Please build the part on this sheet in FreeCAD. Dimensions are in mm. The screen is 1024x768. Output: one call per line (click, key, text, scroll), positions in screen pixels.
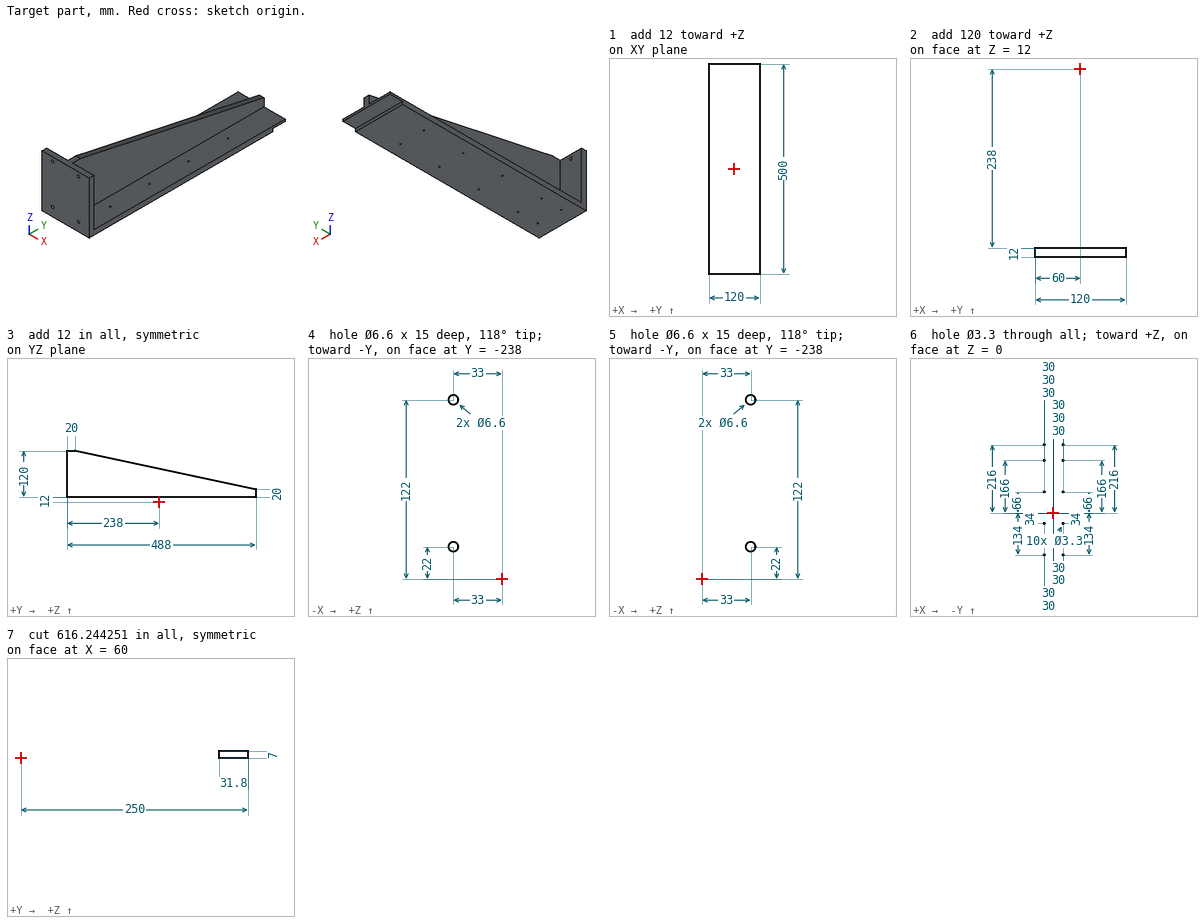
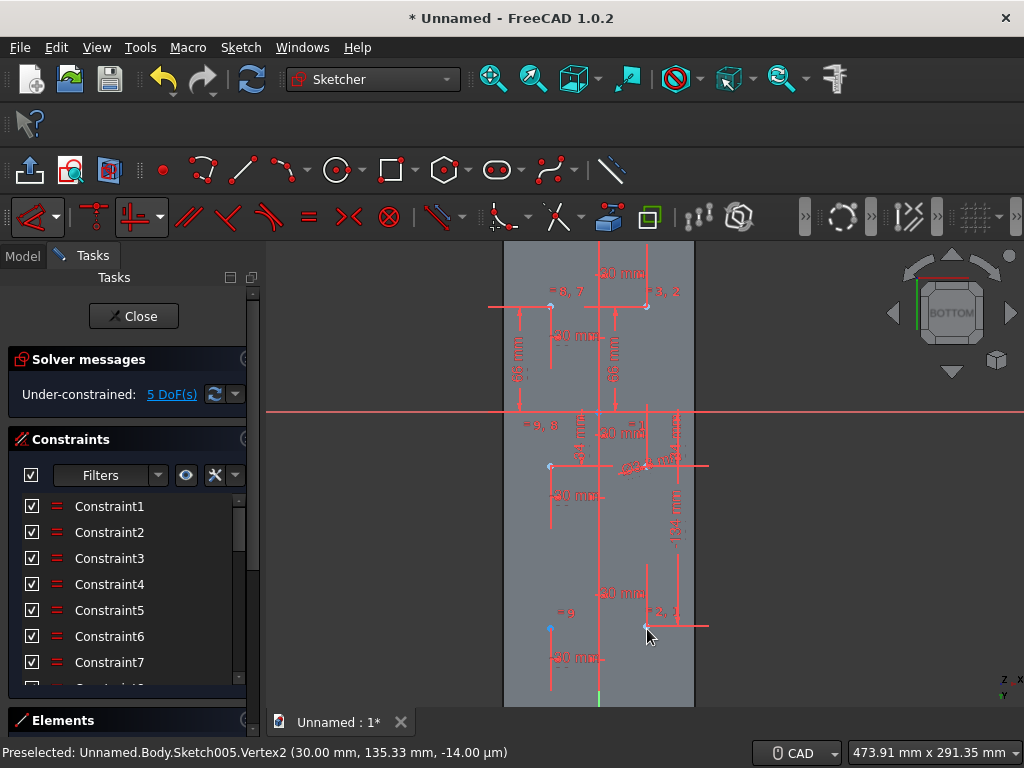
scroll(550, 629, down, 3)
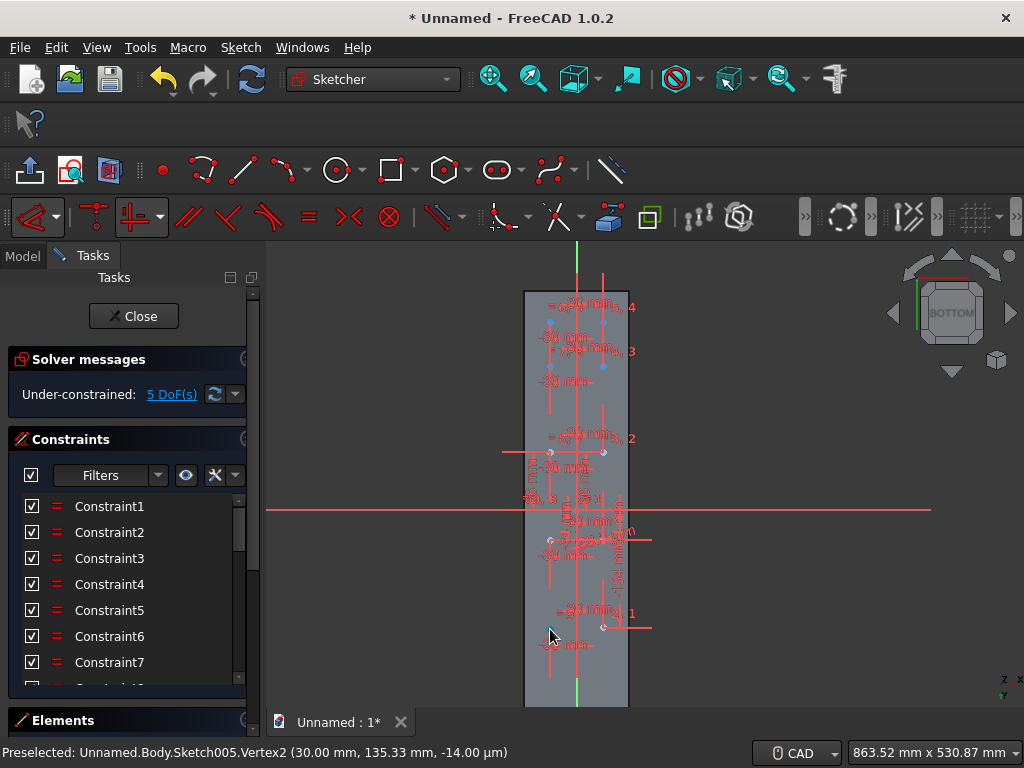
click(603, 366)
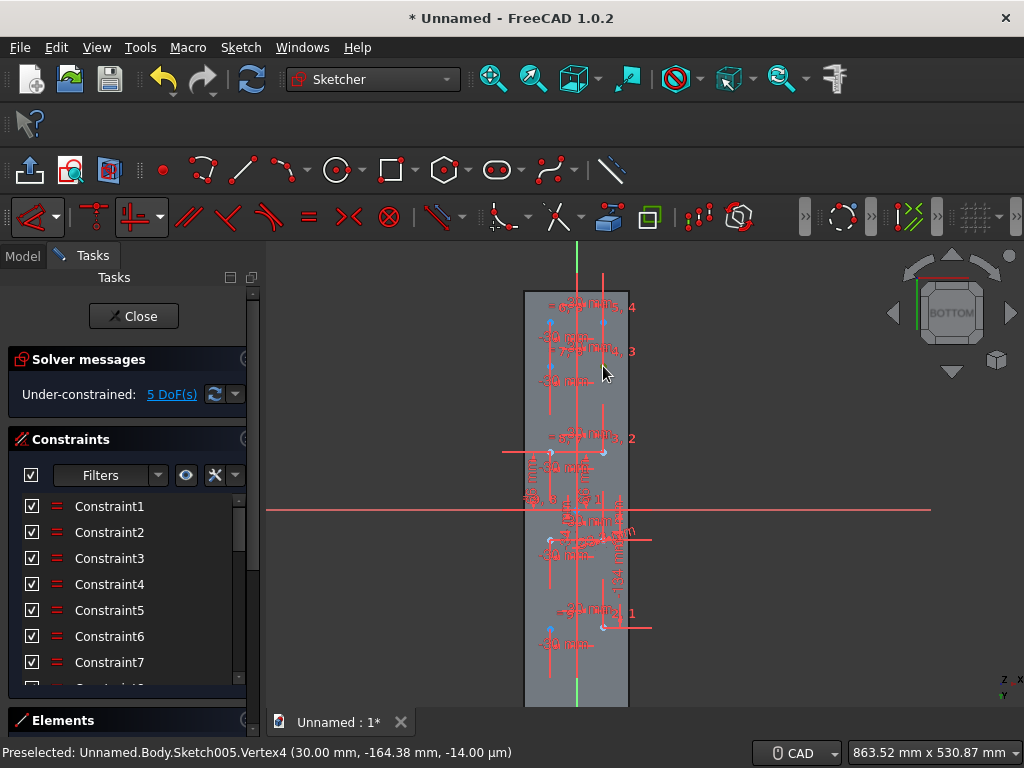
click(58, 218)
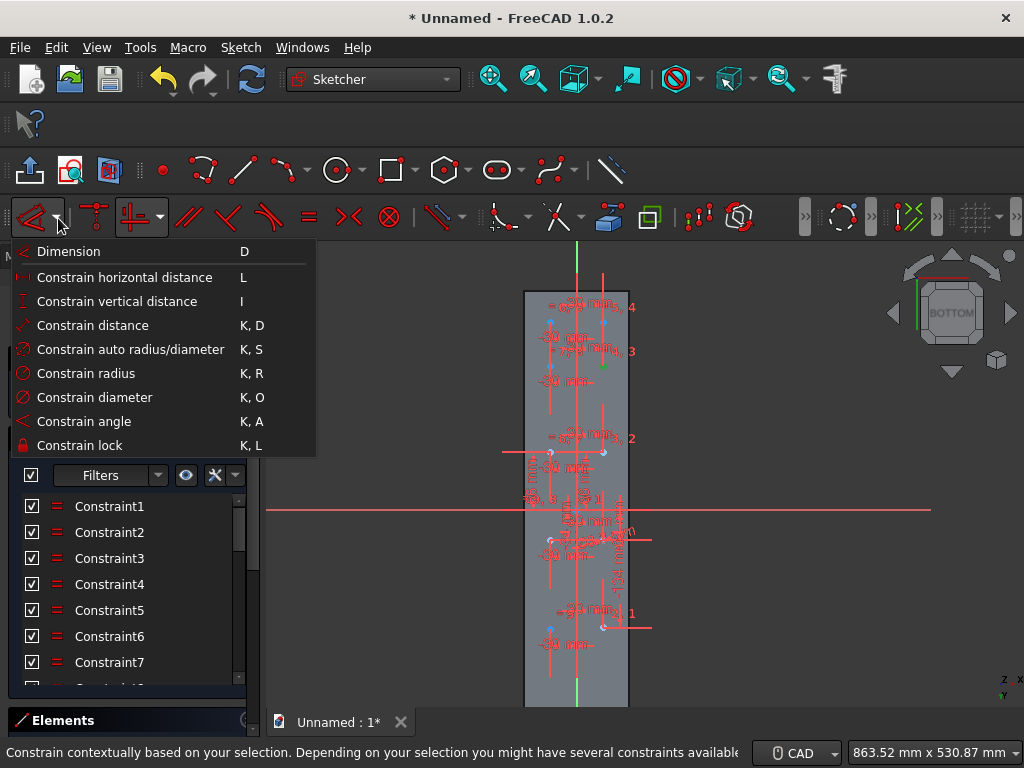
click(164, 301)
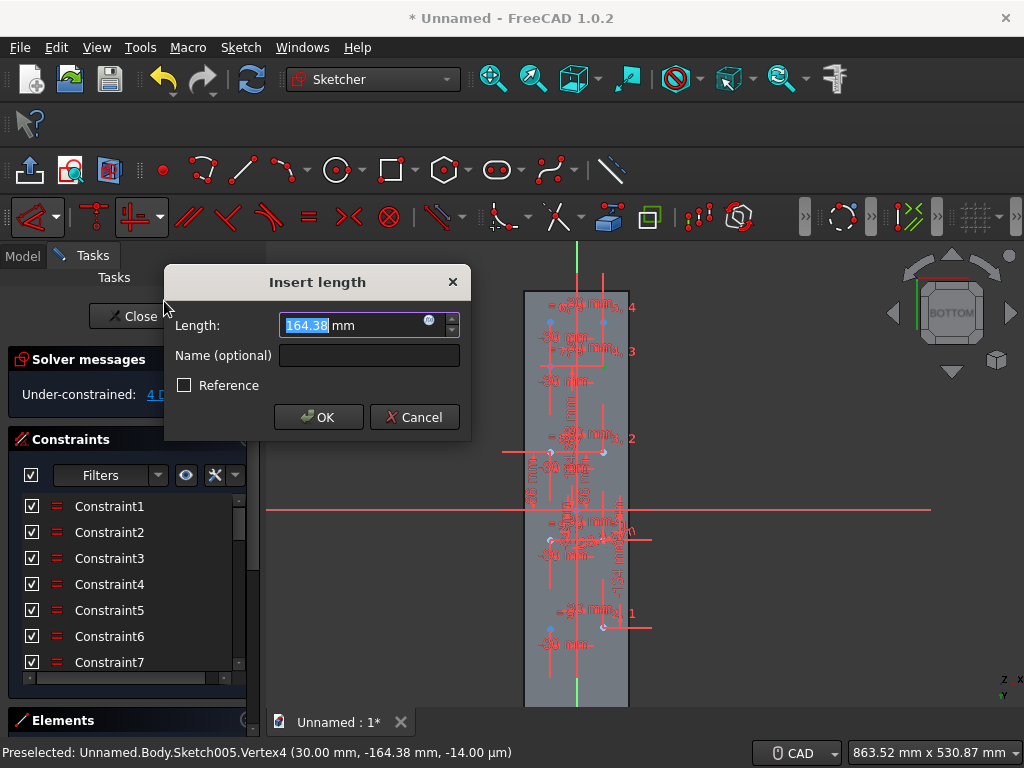
text(166)
key(Return)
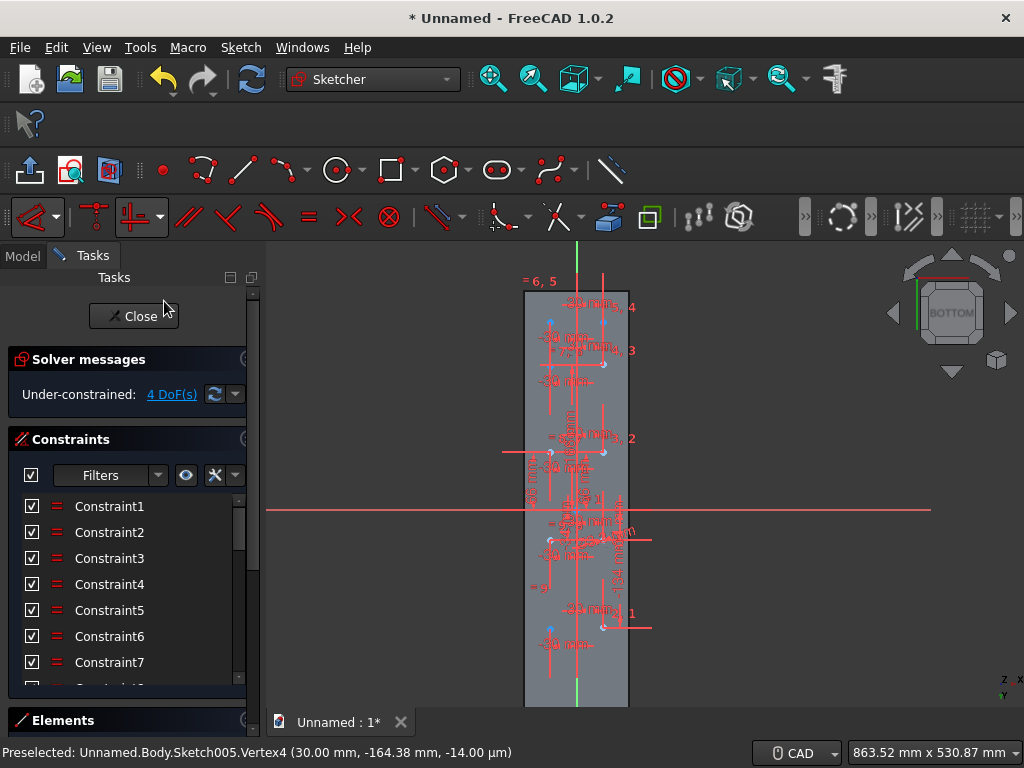
click(603, 322)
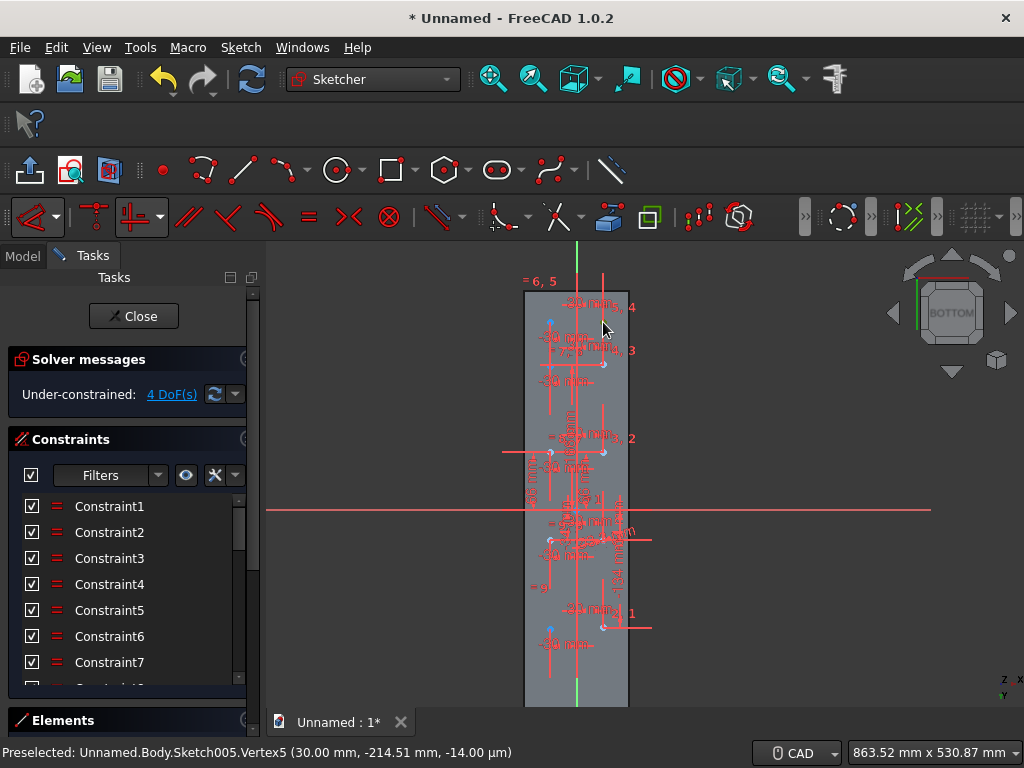
click(58, 218)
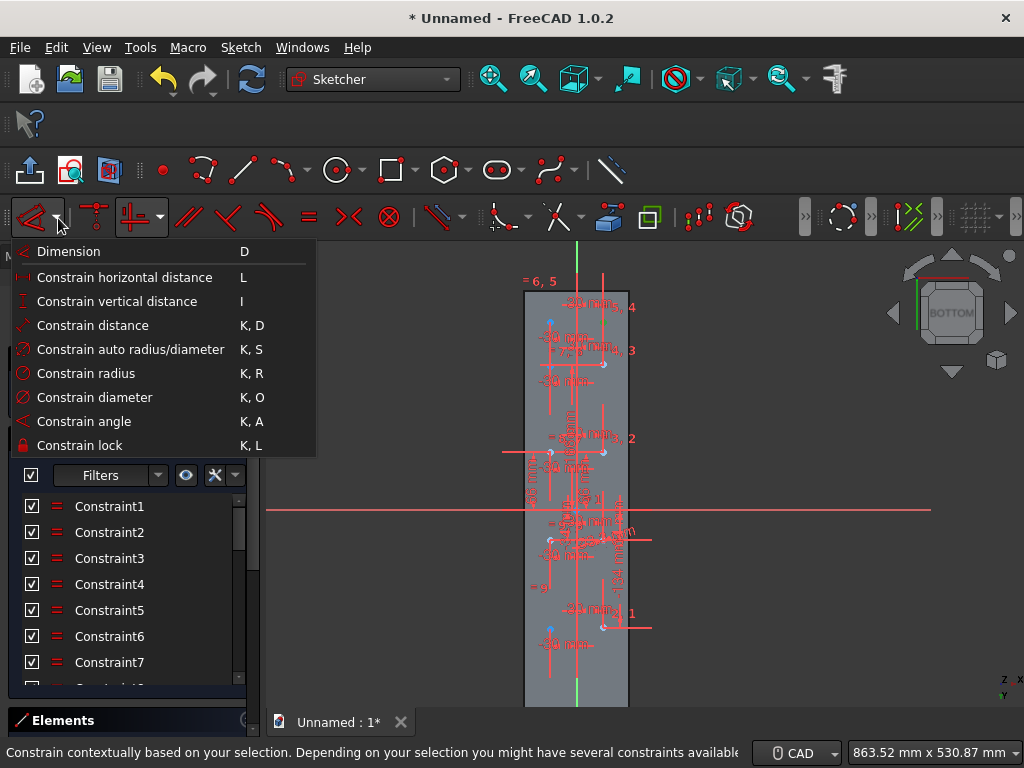
click(164, 301)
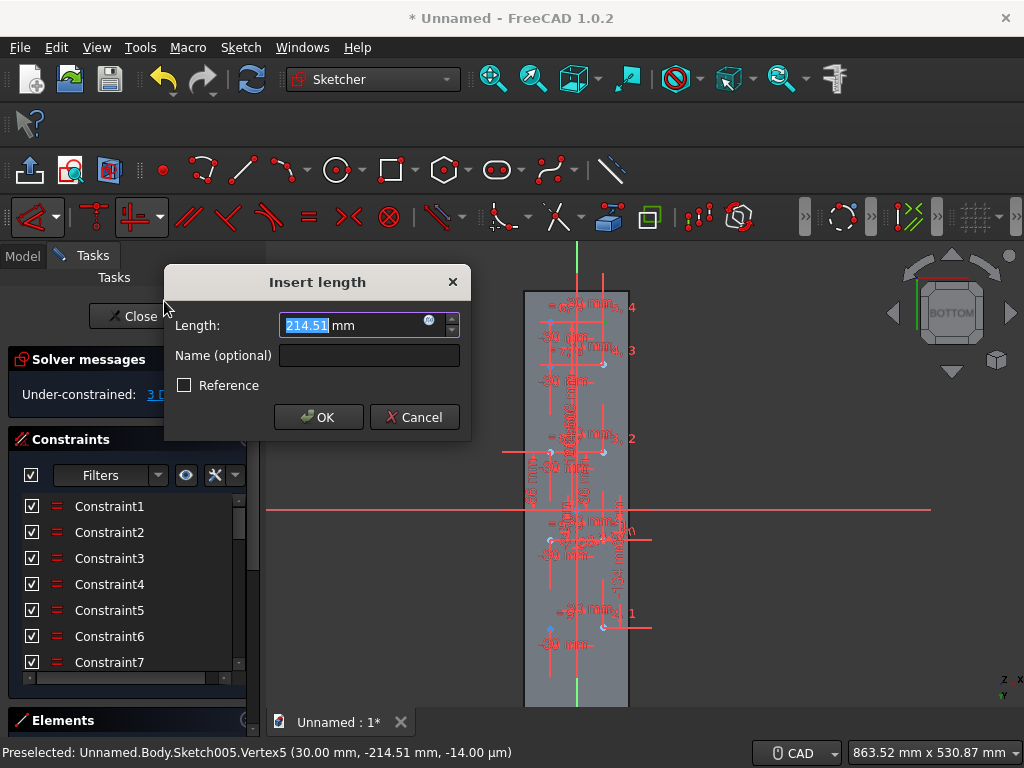
text(216)
key(Return)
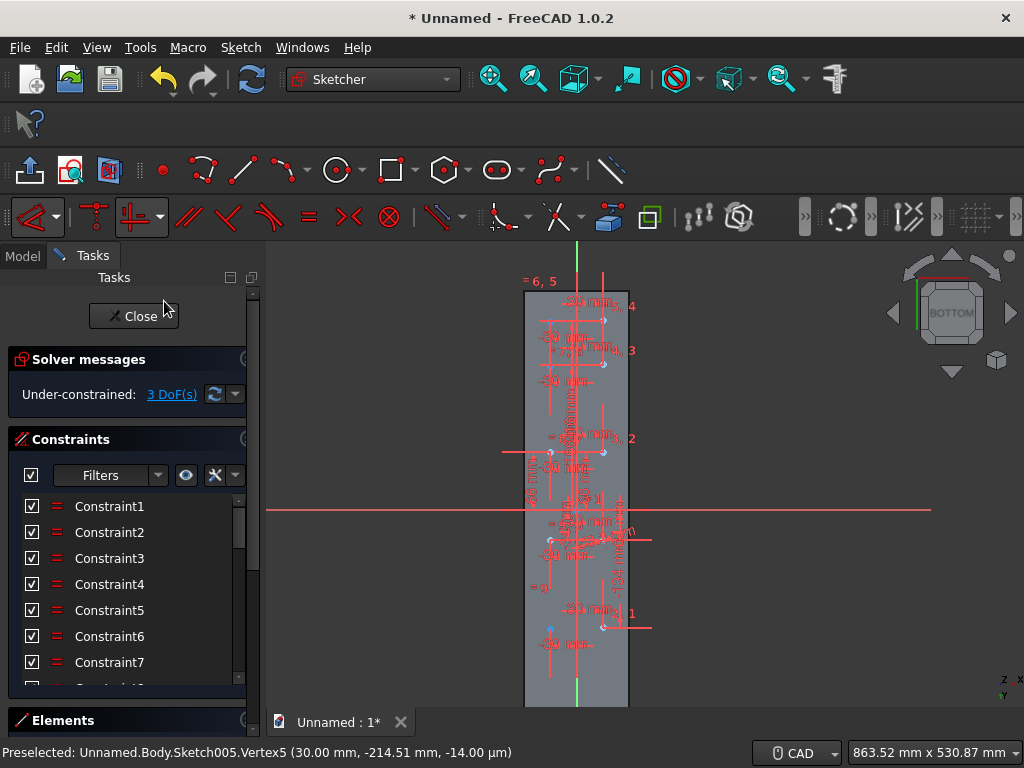
click(550, 322)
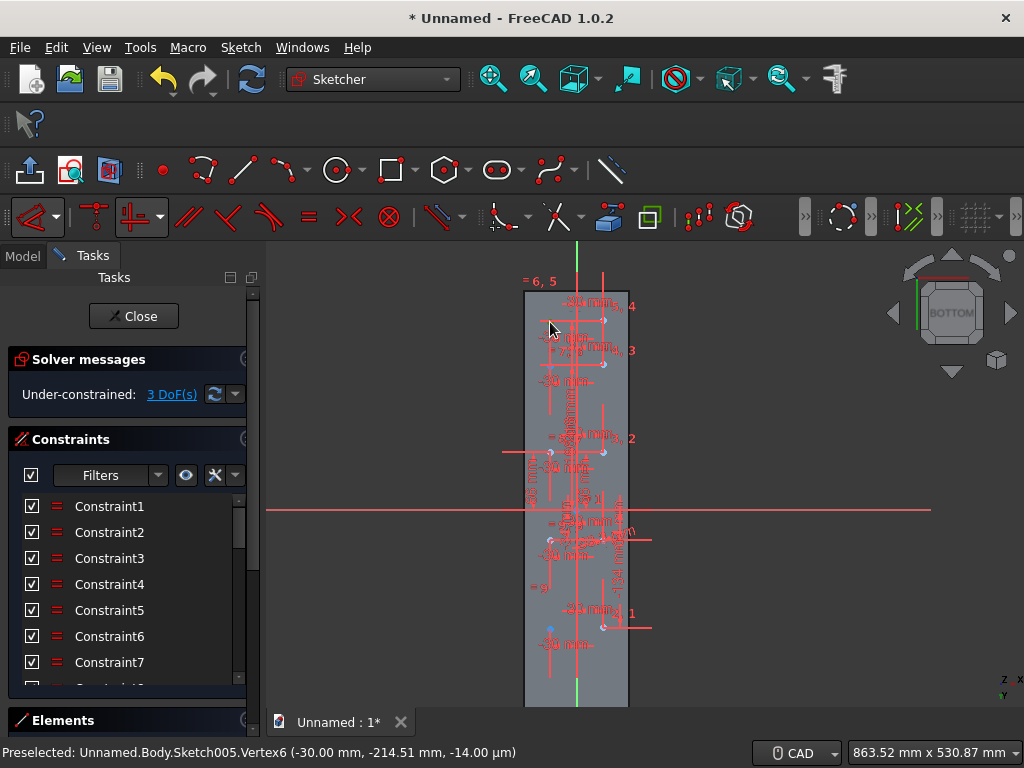
key(i)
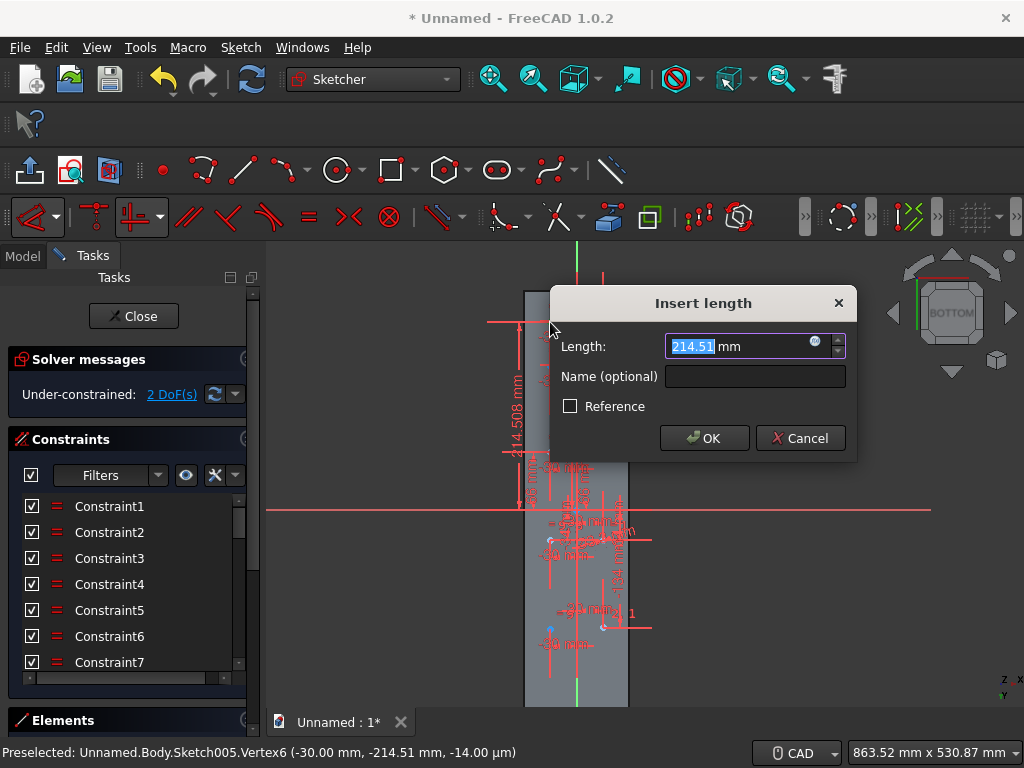
text(216)
key(Return)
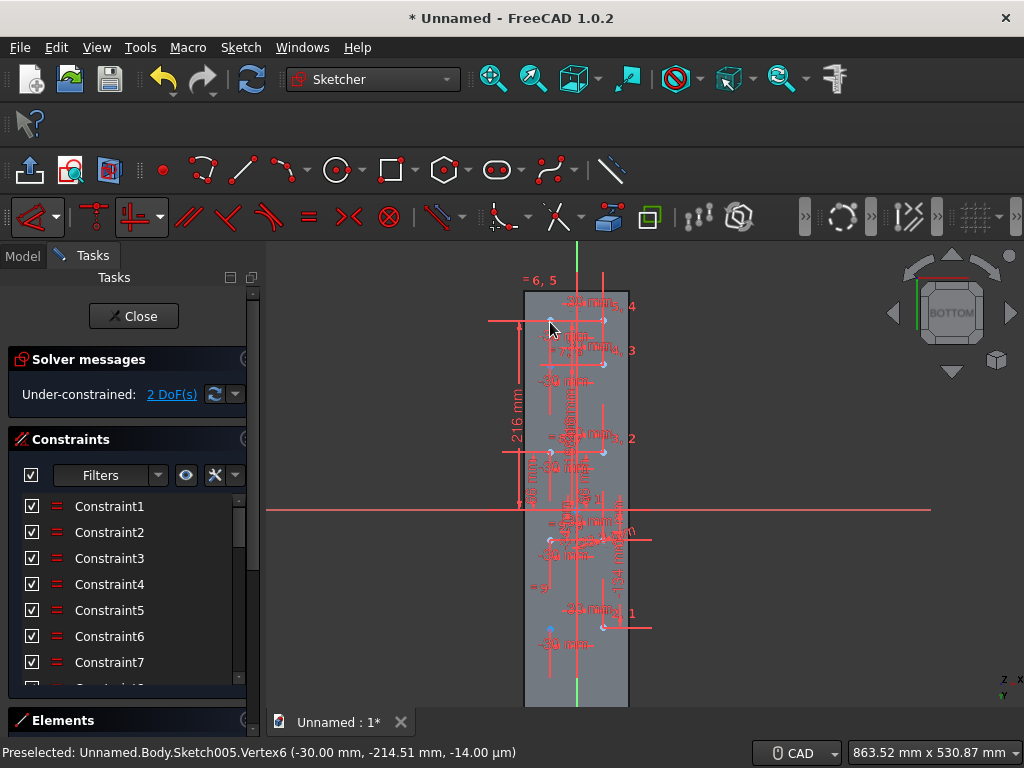
click(550, 366)